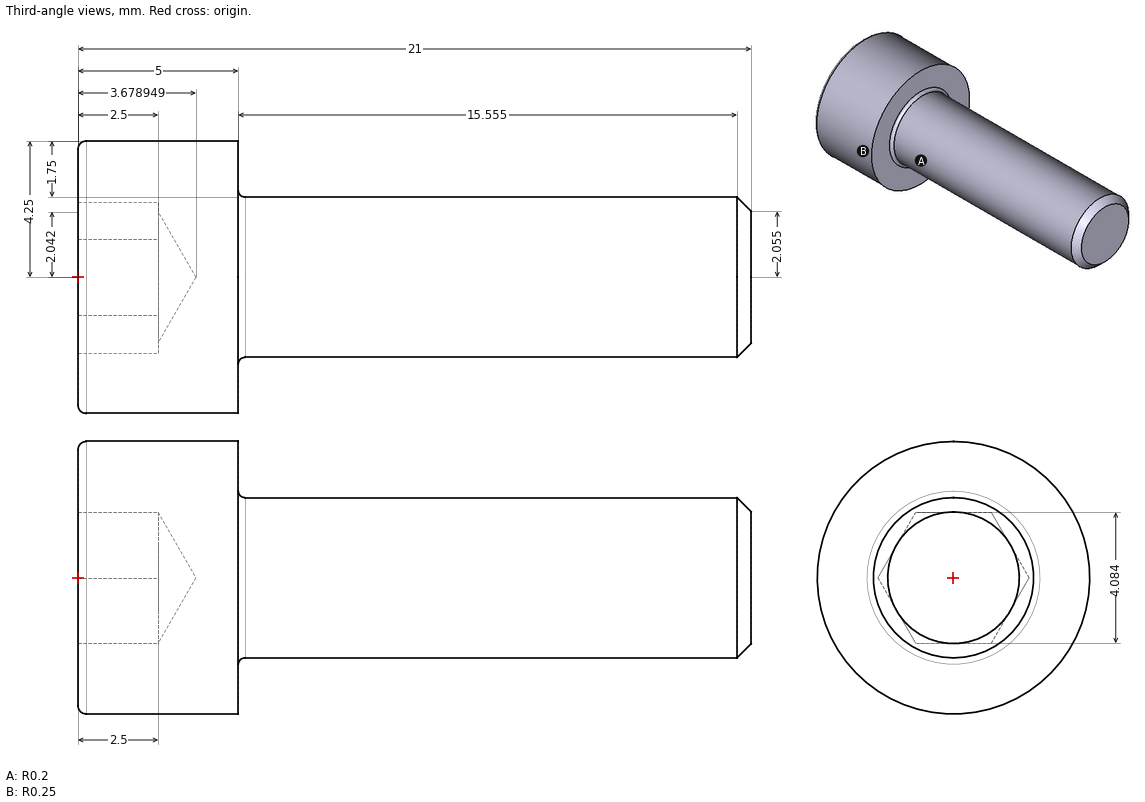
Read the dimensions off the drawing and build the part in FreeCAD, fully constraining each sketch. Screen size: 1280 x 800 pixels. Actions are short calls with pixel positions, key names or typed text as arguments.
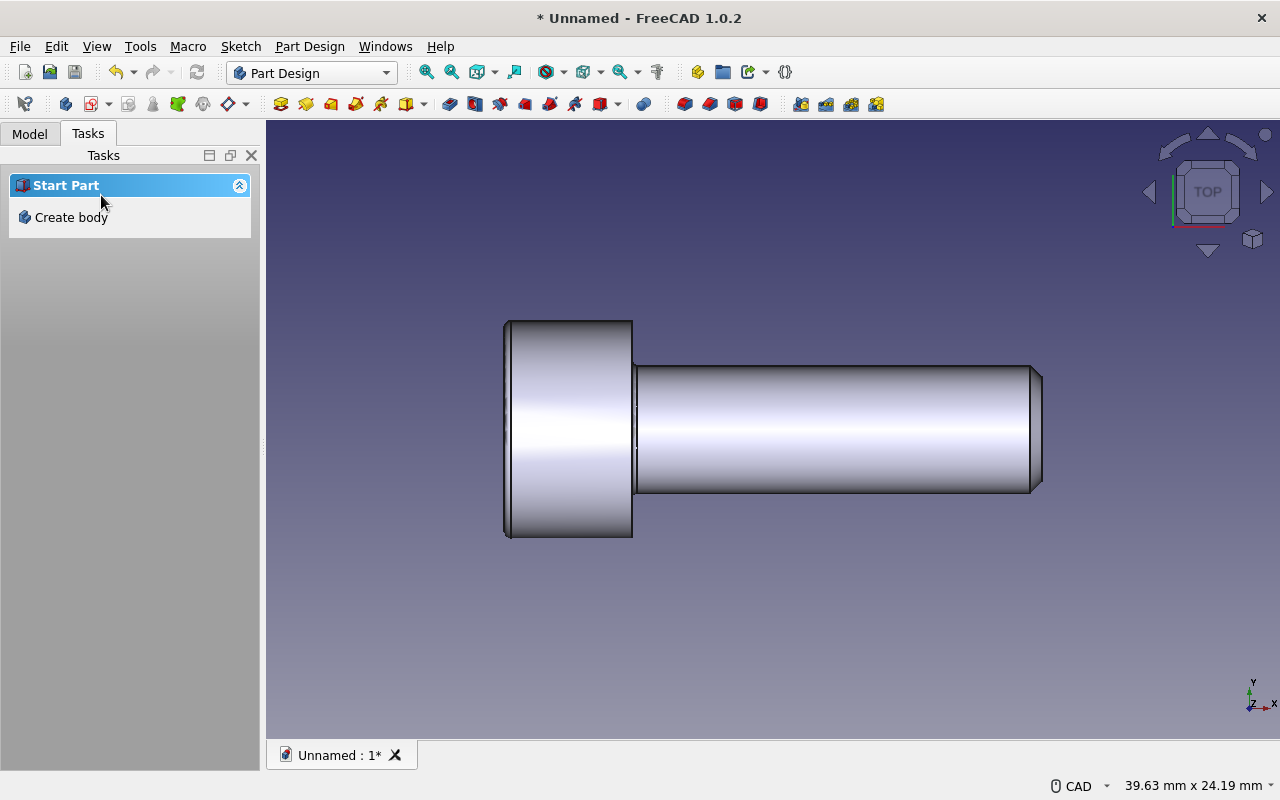
click(90, 104)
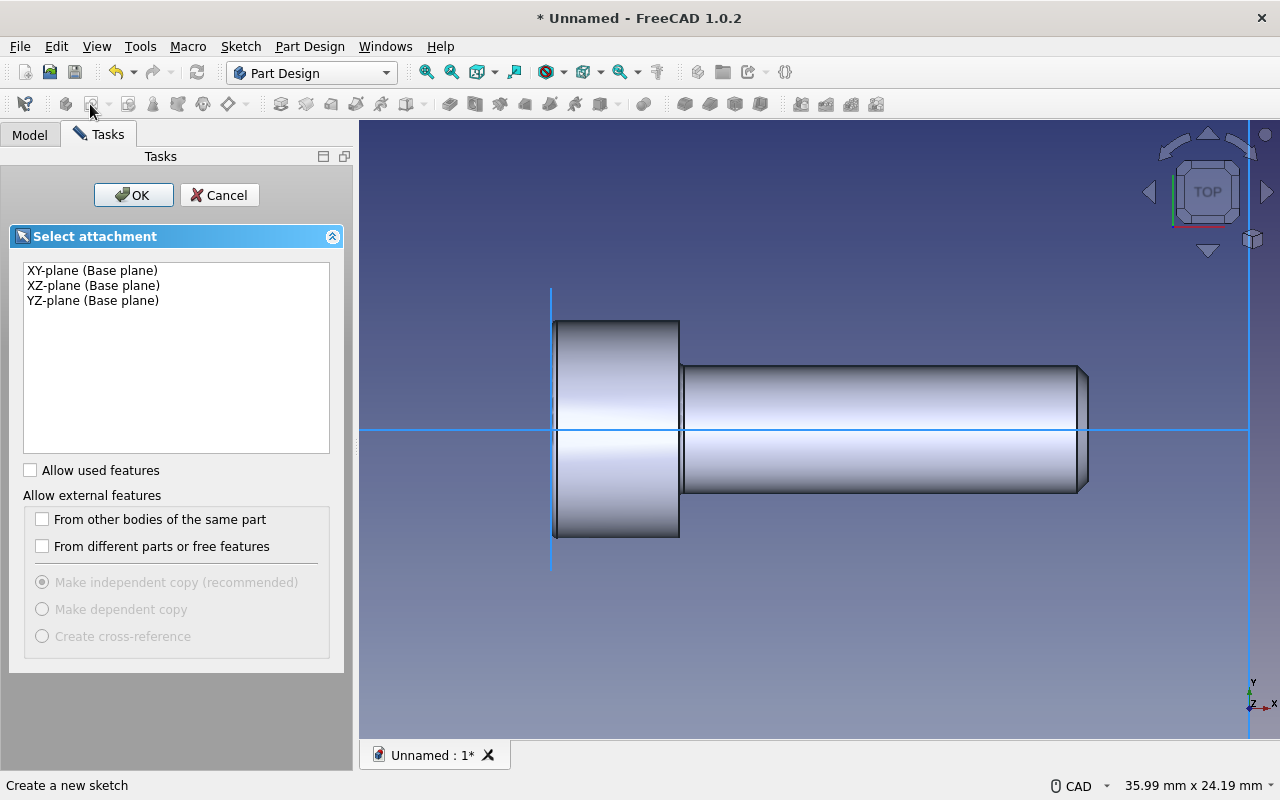
click(84, 270)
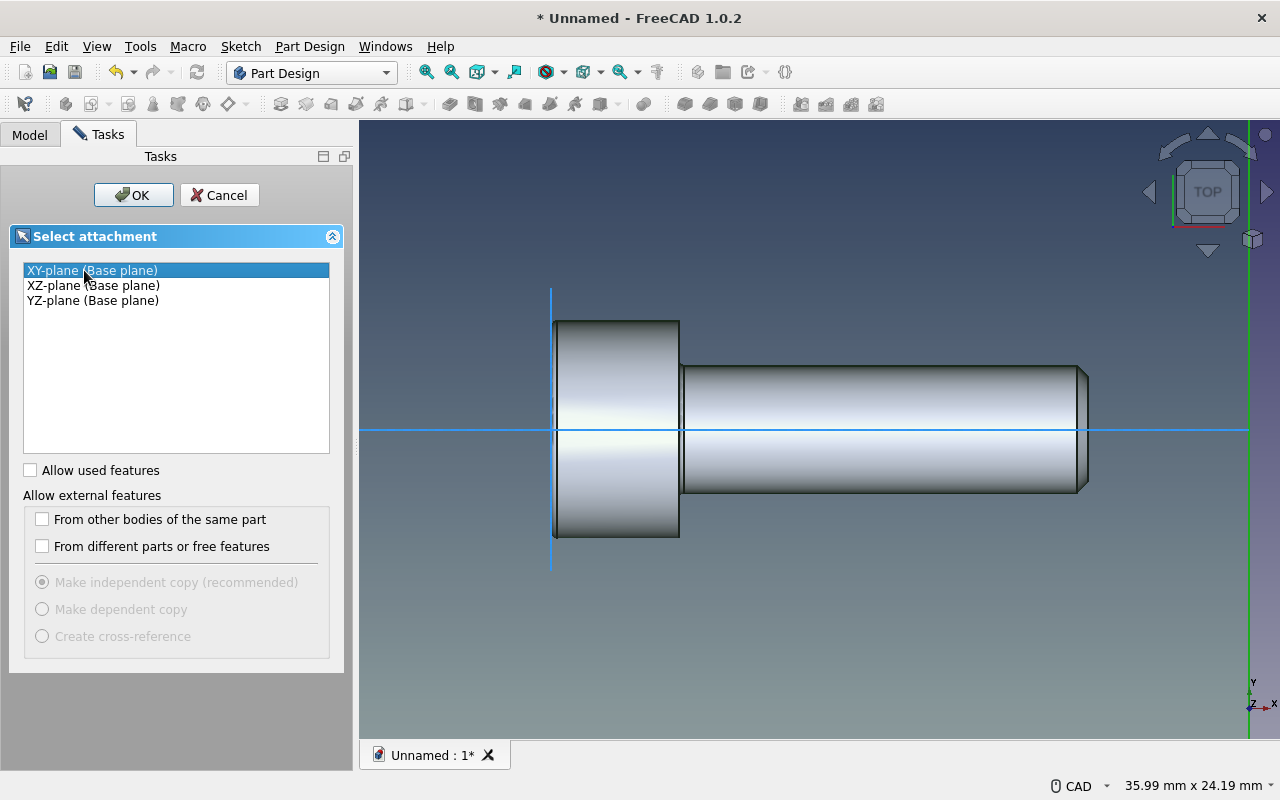
click(134, 195)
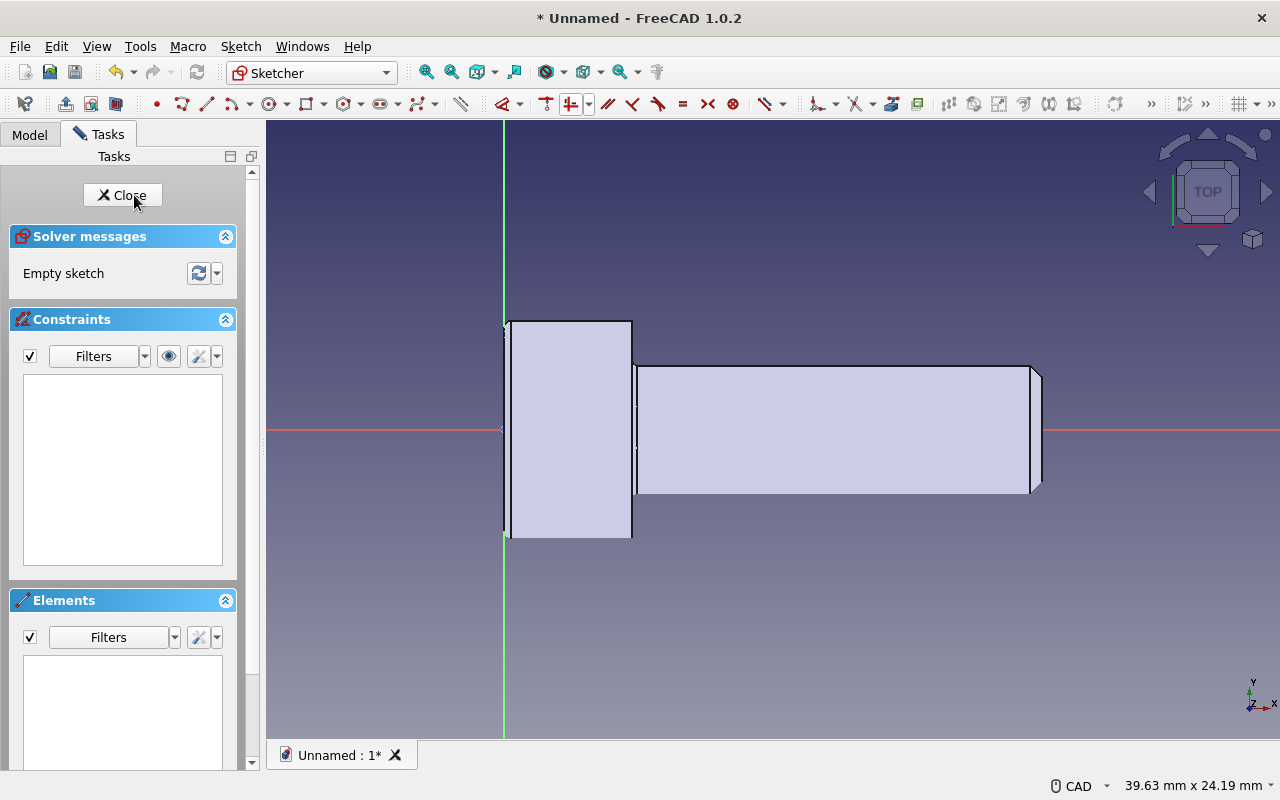
click(116, 104)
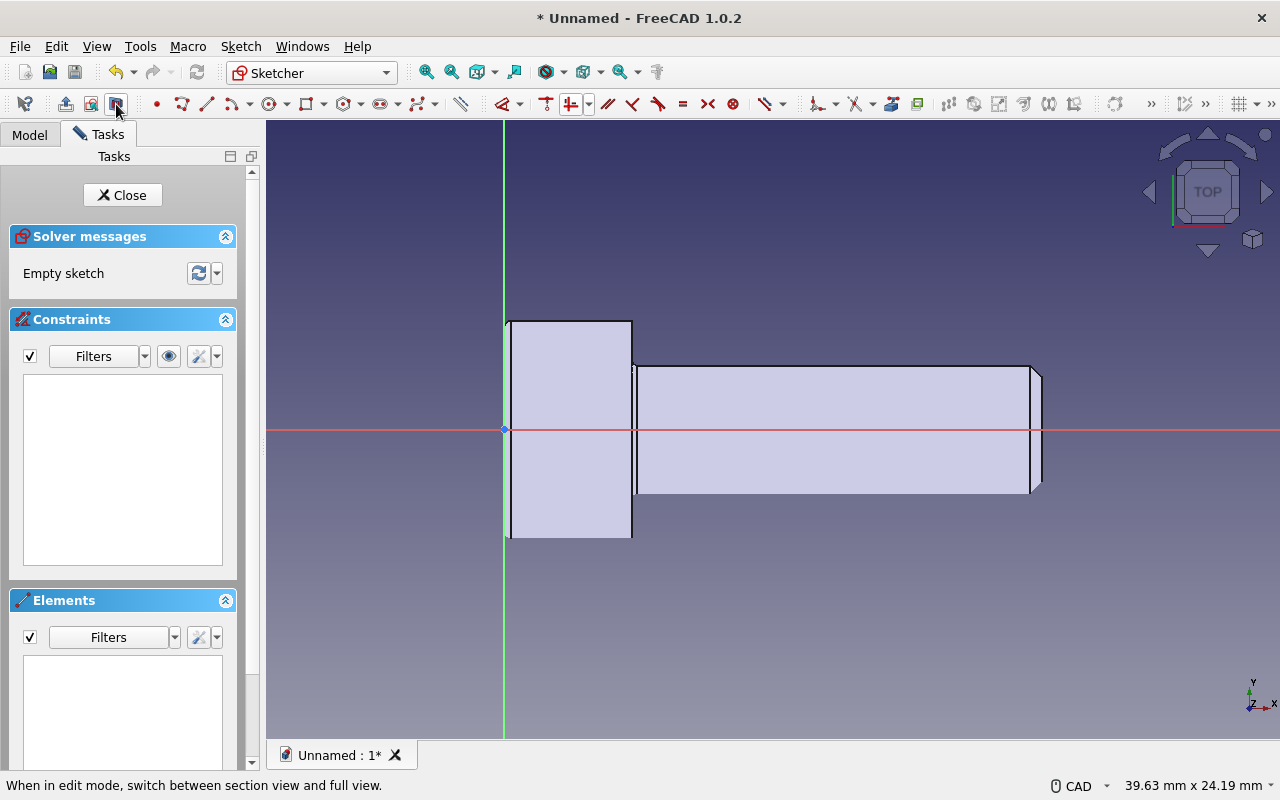
scroll(521, 398, up, 9)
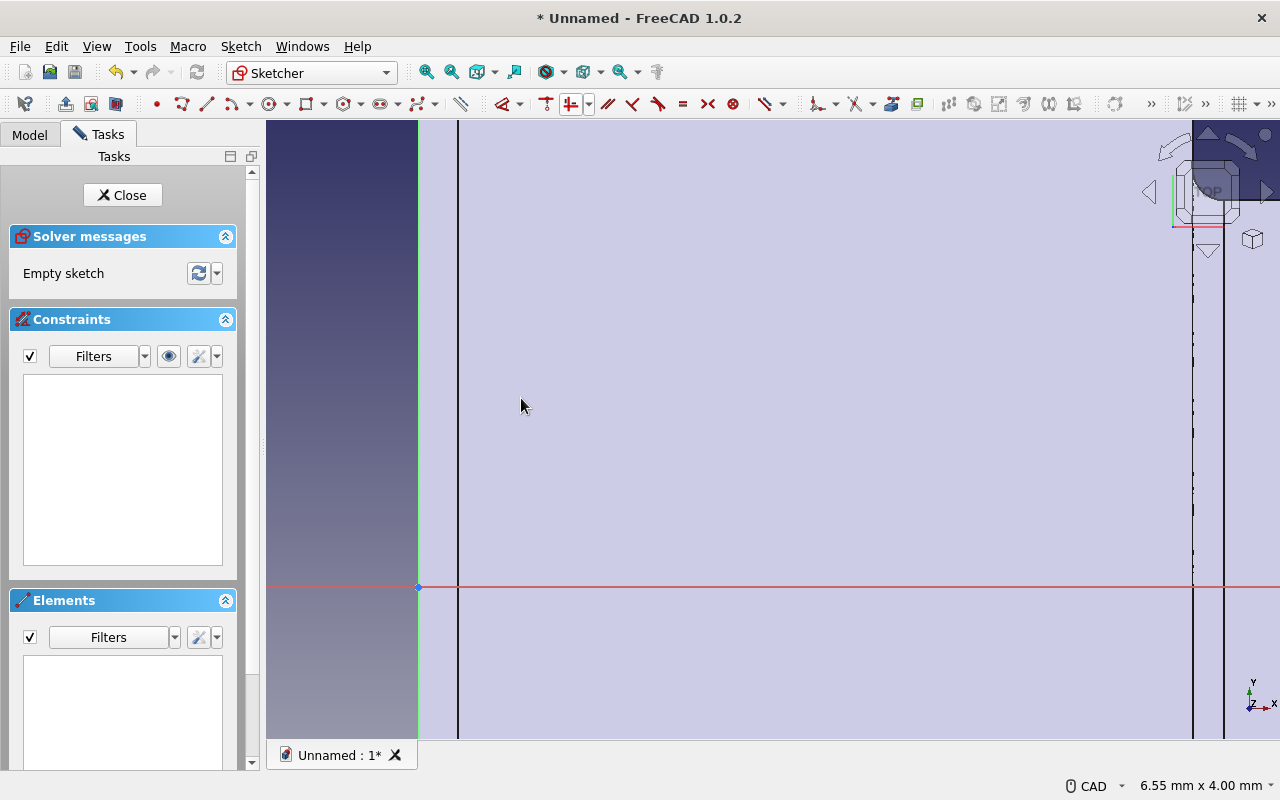
click(182, 104)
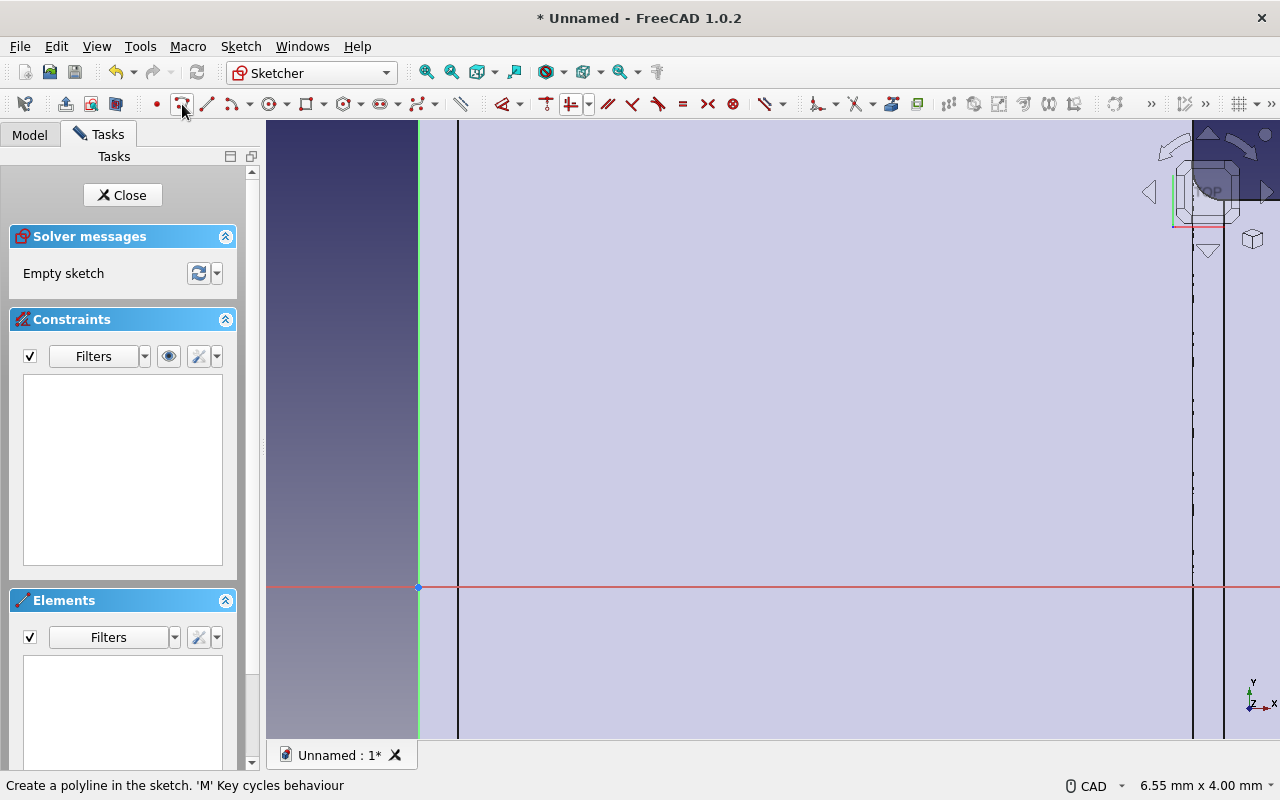
click(419, 587)
click(988, 578)
click(806, 271)
click(428, 271)
click(419, 587)
key(Escape)
key(Escape)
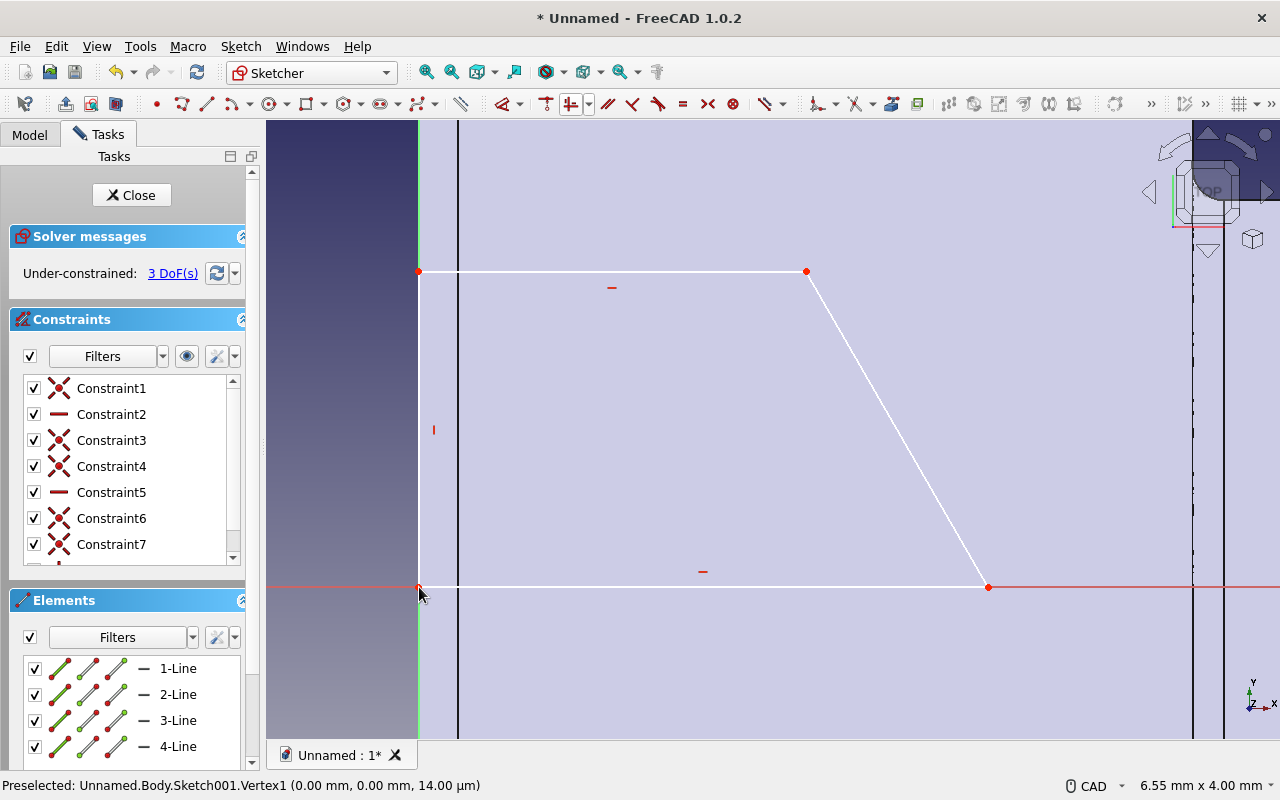
click(502, 104)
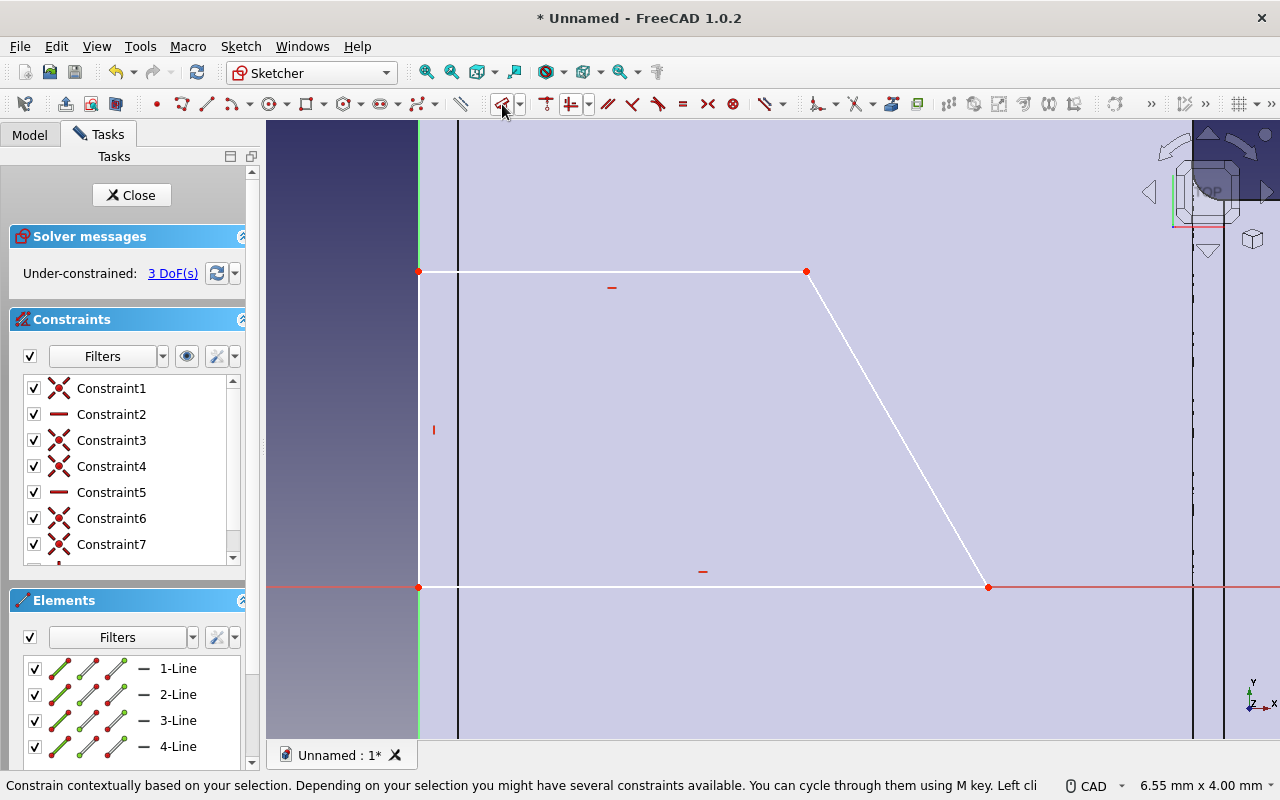
click(690, 272)
click(612, 238)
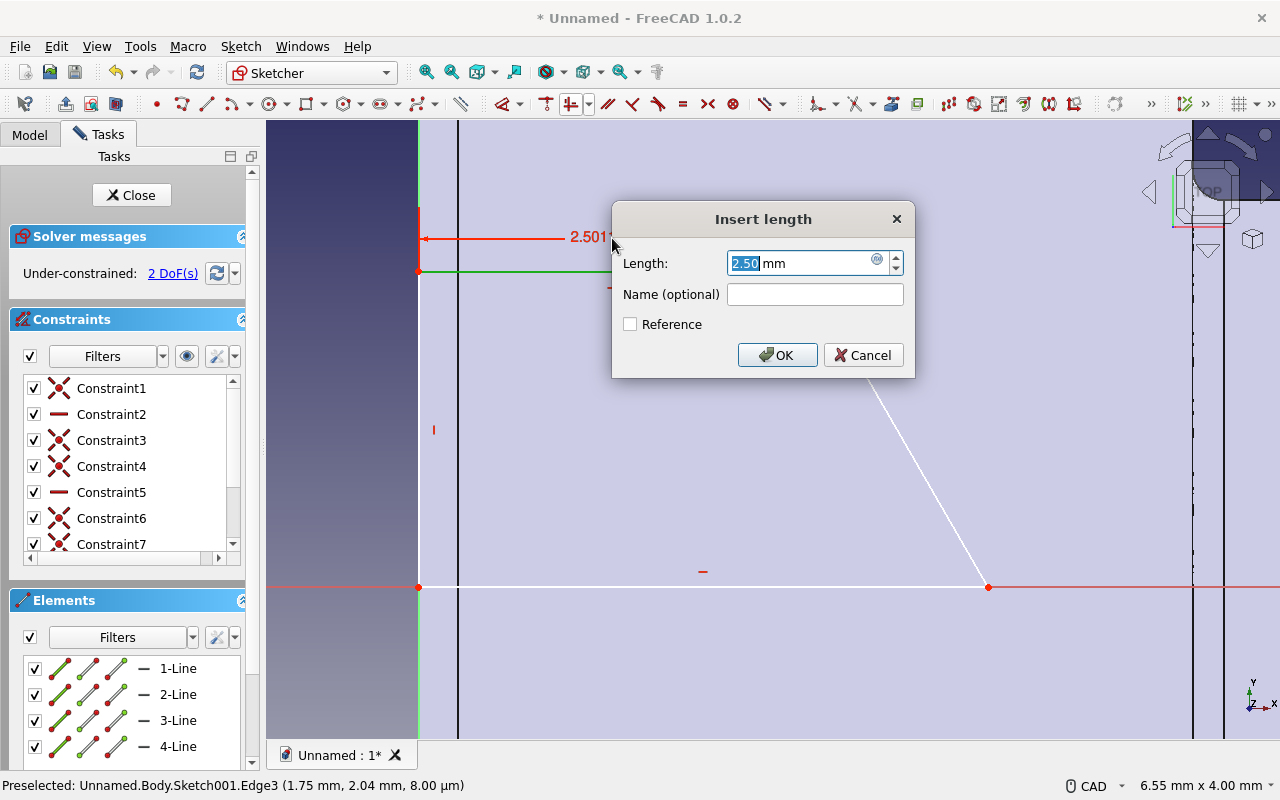
text(2.5)
key(Return)